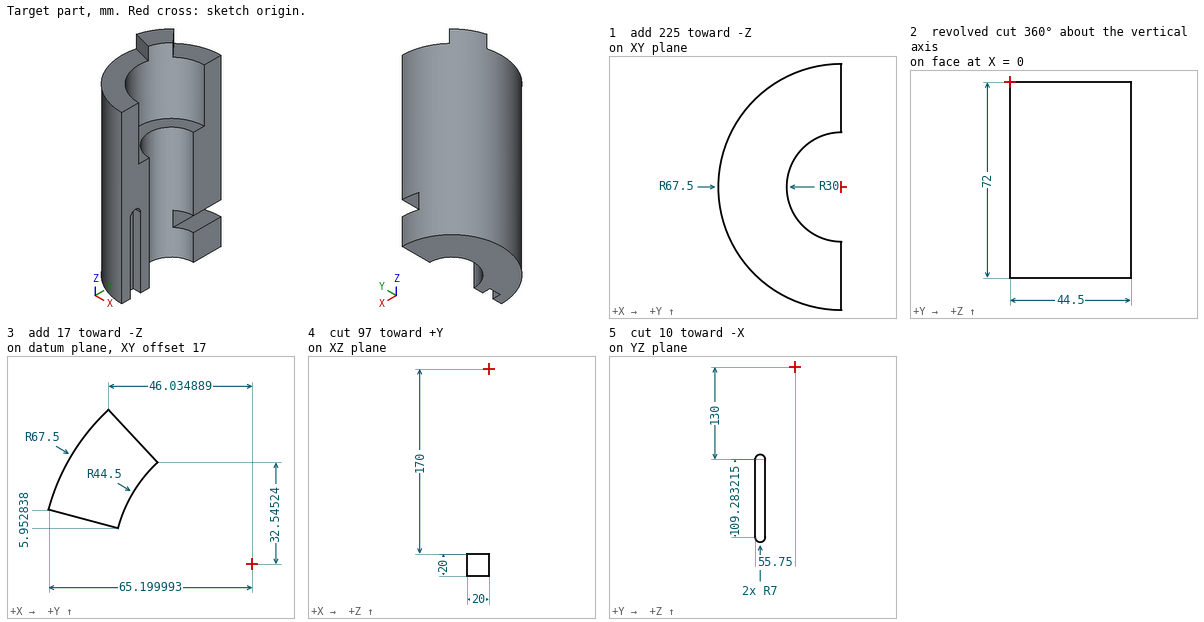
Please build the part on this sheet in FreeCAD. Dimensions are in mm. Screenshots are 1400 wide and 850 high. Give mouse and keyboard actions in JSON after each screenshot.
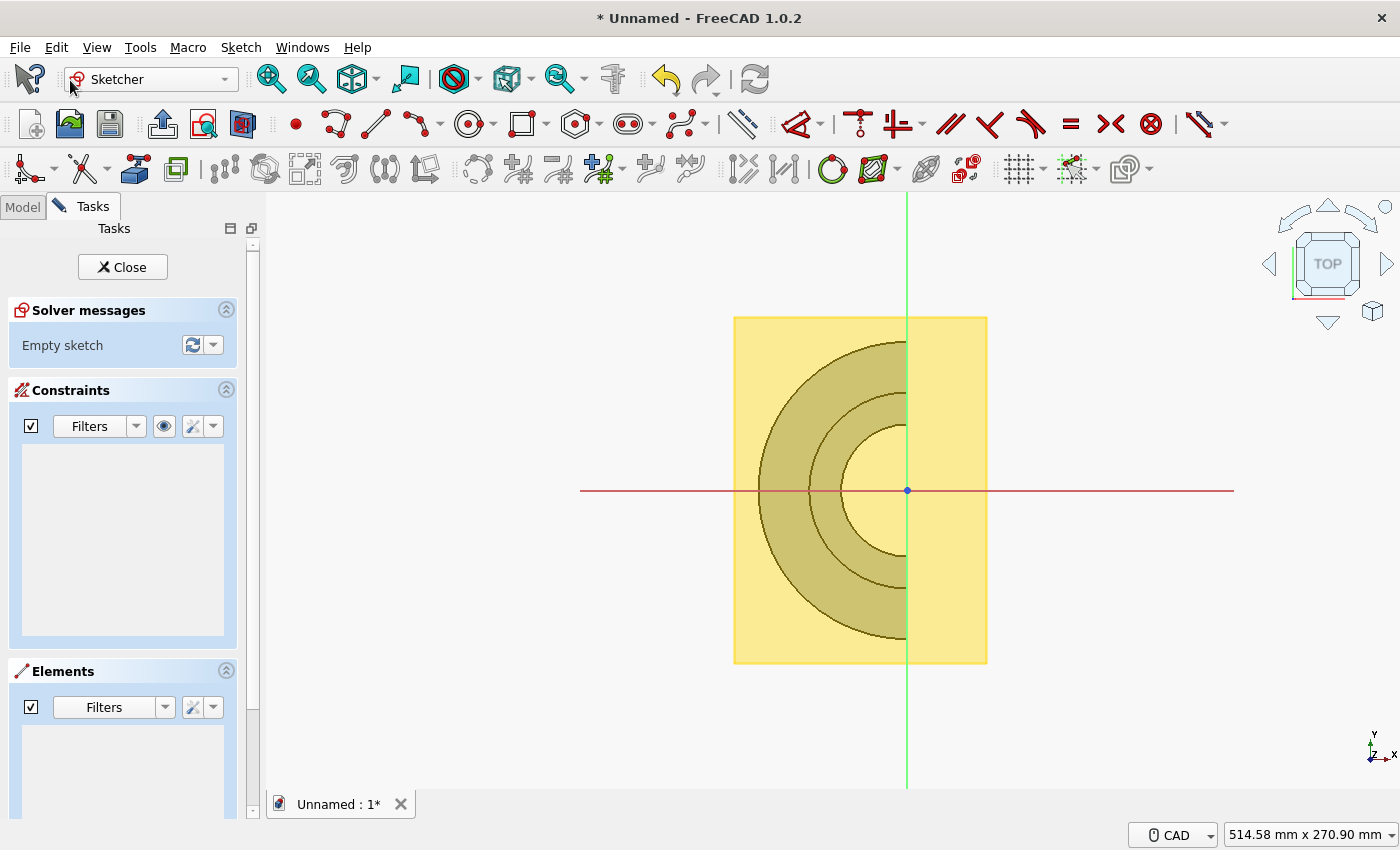
{"action": "scroll", "coordinate": [866, 413], "scroll_direction": "up", "scroll_amount": 6}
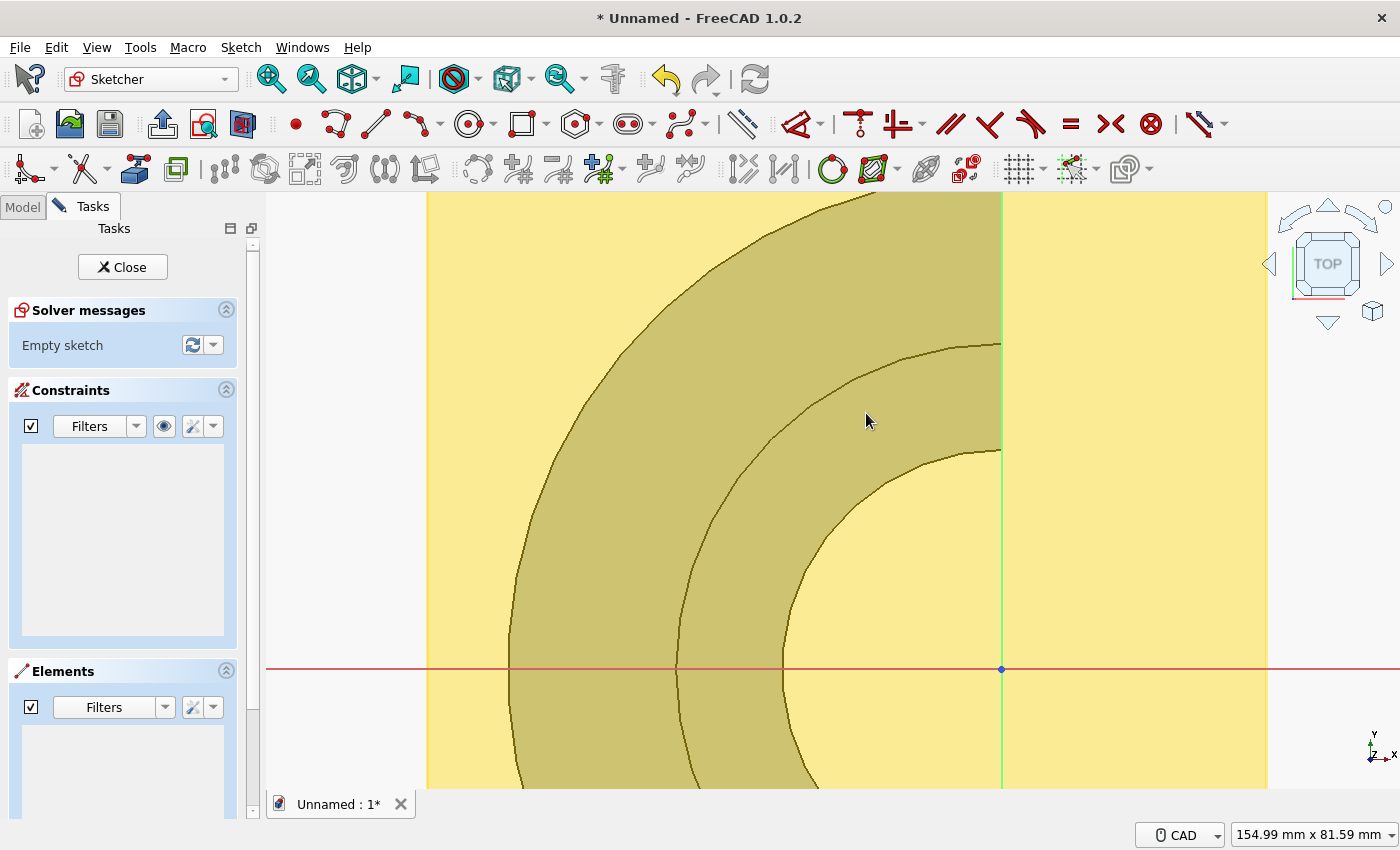
{"action": "key", "text": "g l"}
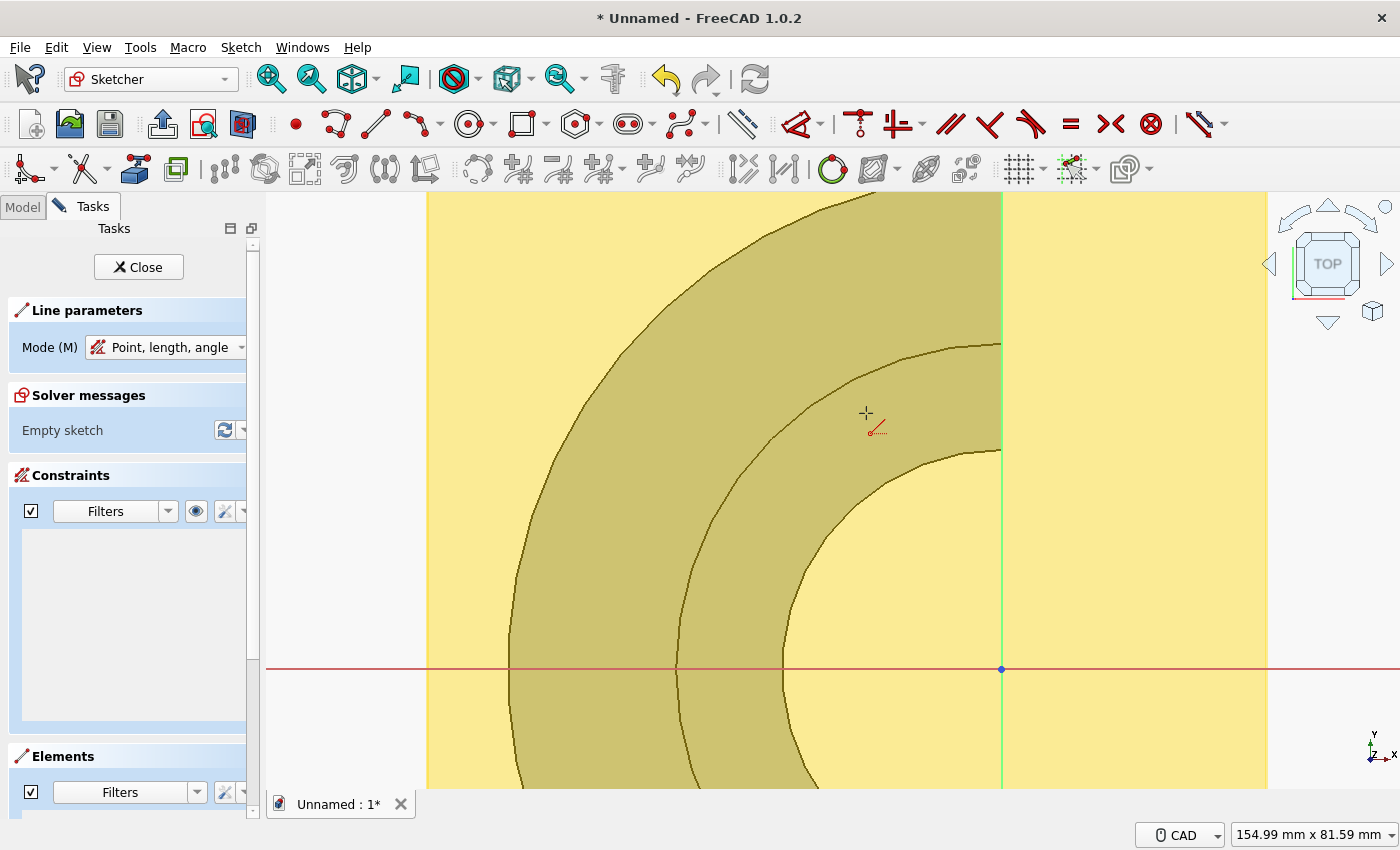
{"action": "left_click", "coordinate": [780, 431]}
{"action": "left_click", "coordinate": [665, 308]}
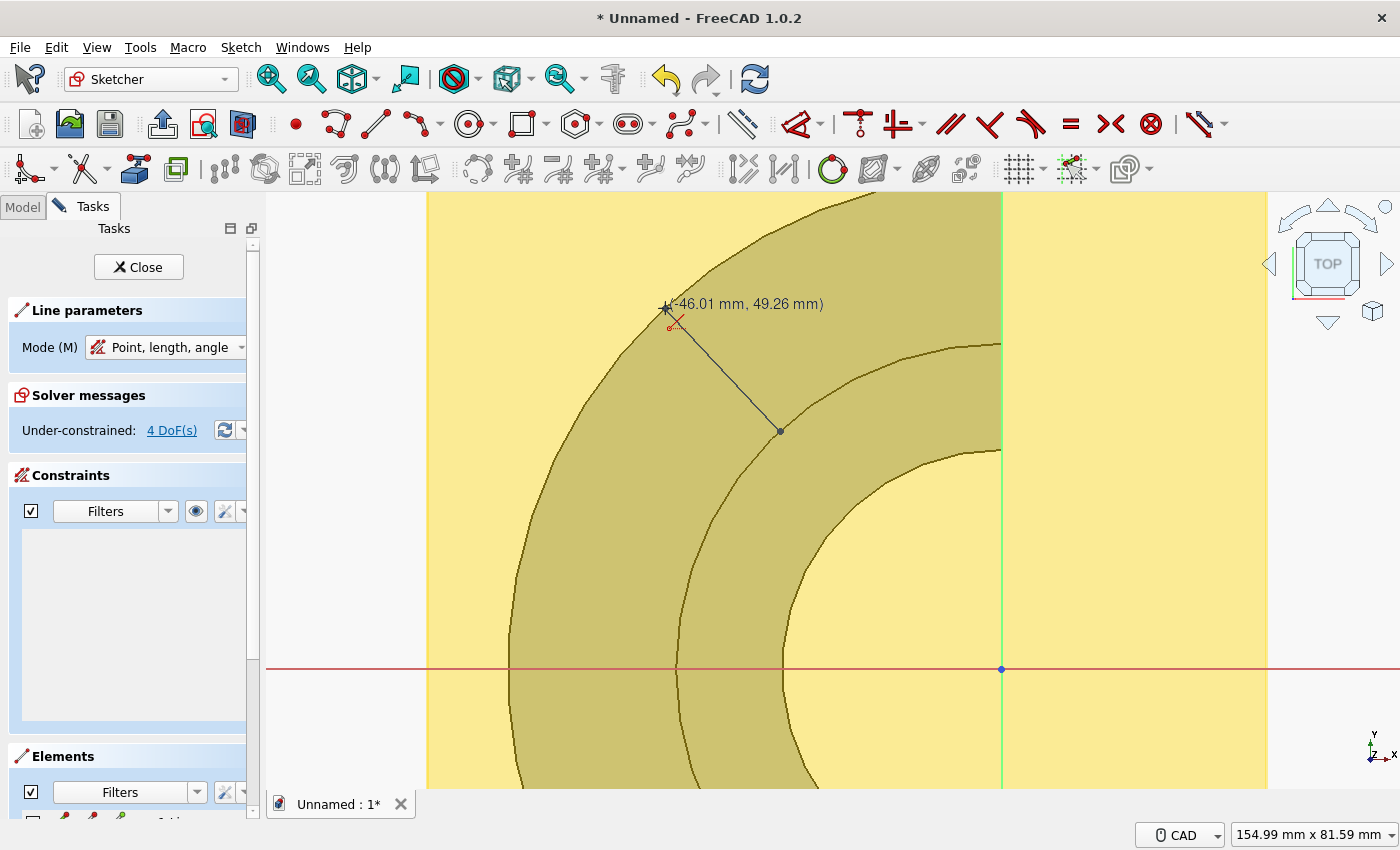
{"action": "left_click", "coordinate": [525, 542]}
{"action": "left_click", "coordinate": [687, 585]}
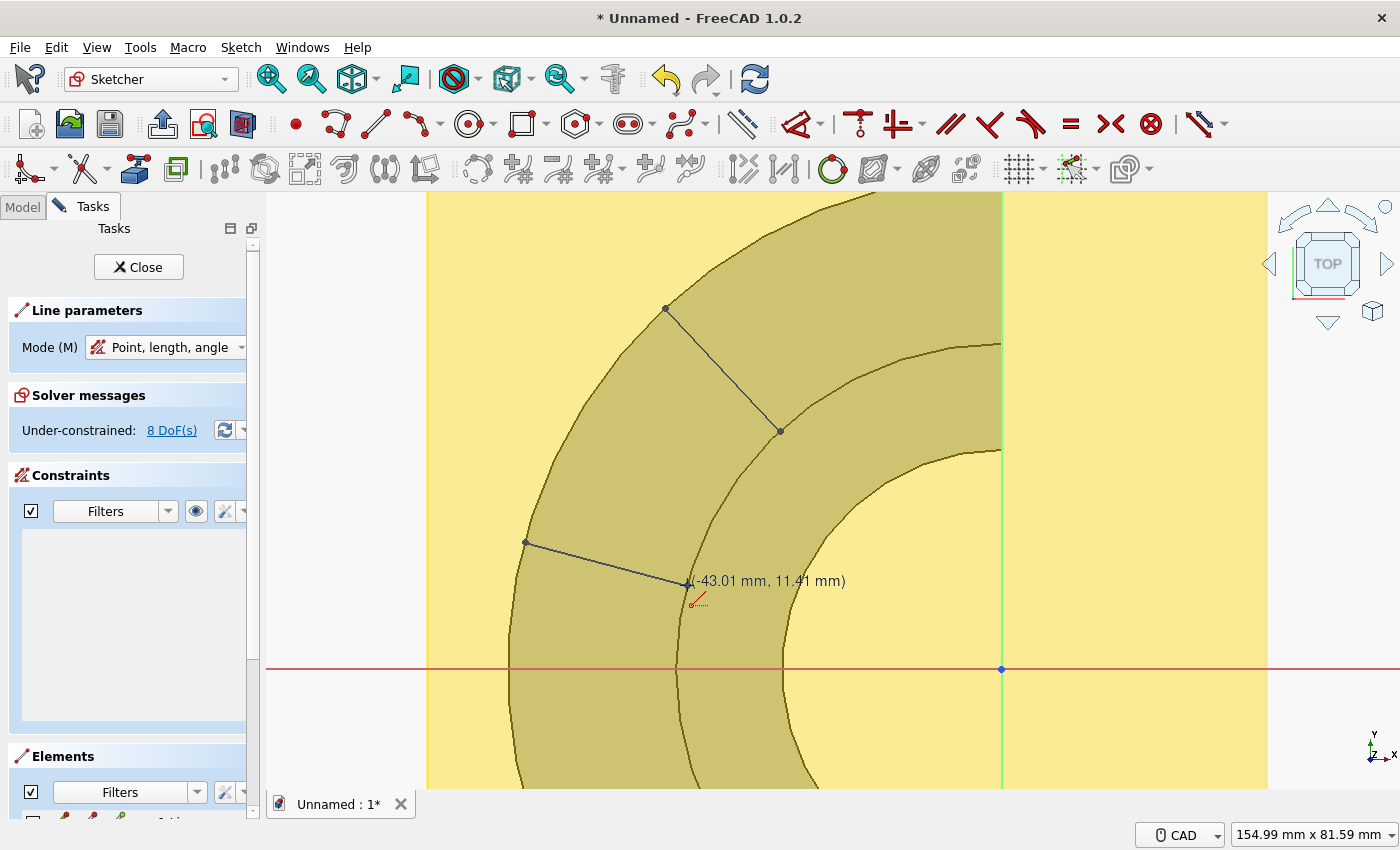
{"action": "key", "text": "g 3 a"}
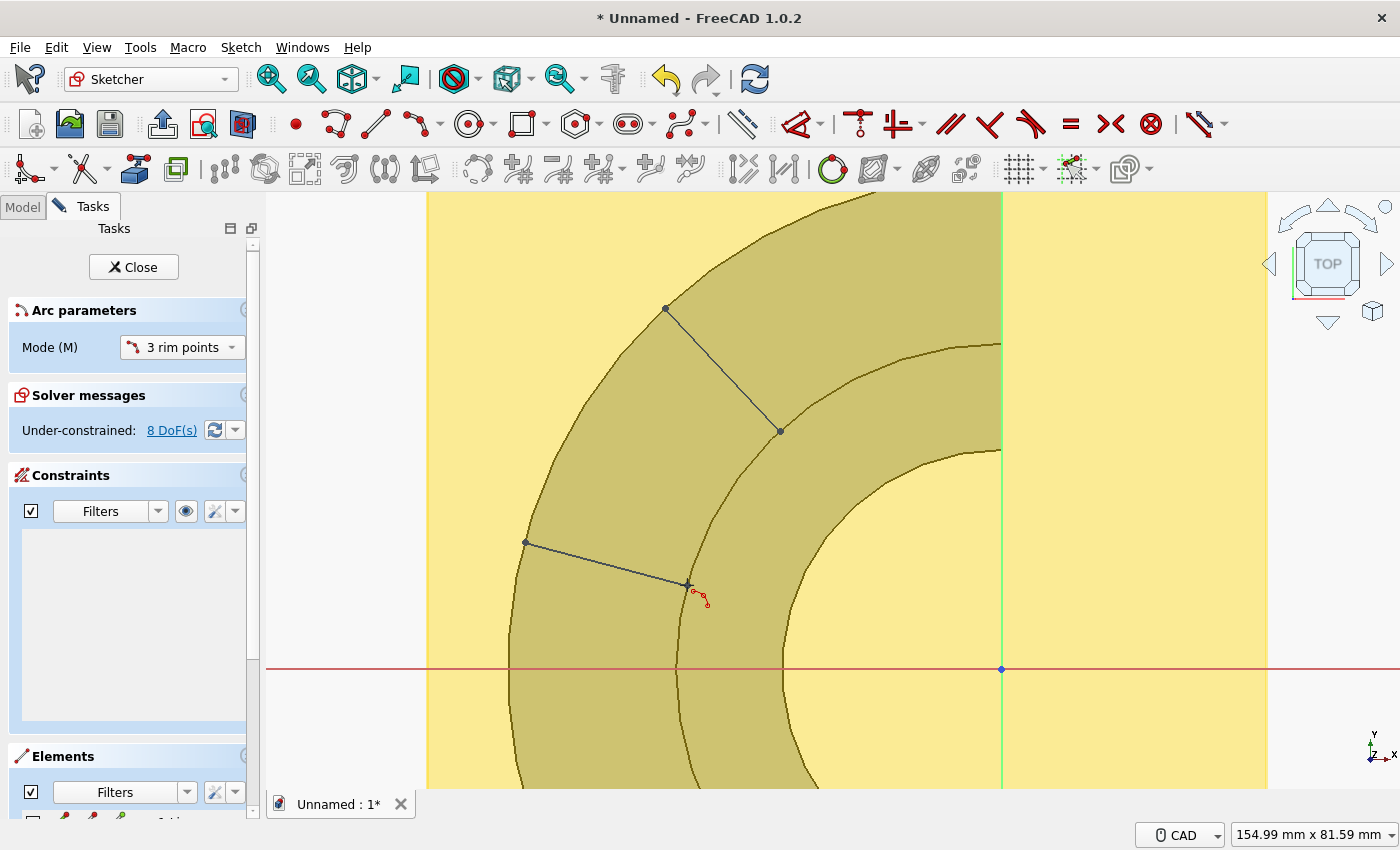
{"action": "left_click", "coordinate": [665, 309]}
{"action": "left_click", "coordinate": [525, 543]}
{"action": "left_click", "coordinate": [578, 415]}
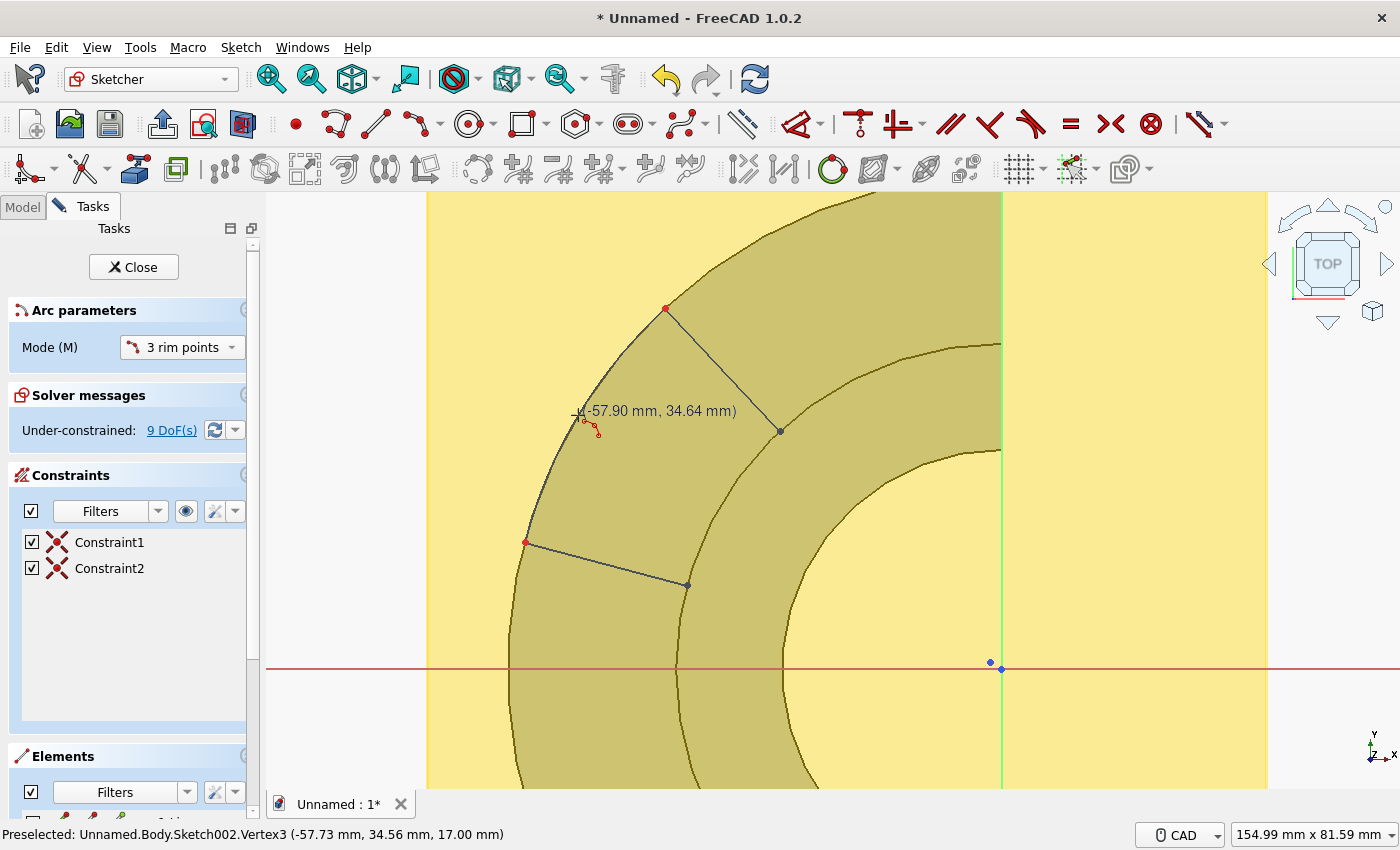
{"action": "left_click", "coordinate": [687, 586]}
{"action": "left_click", "coordinate": [780, 432]}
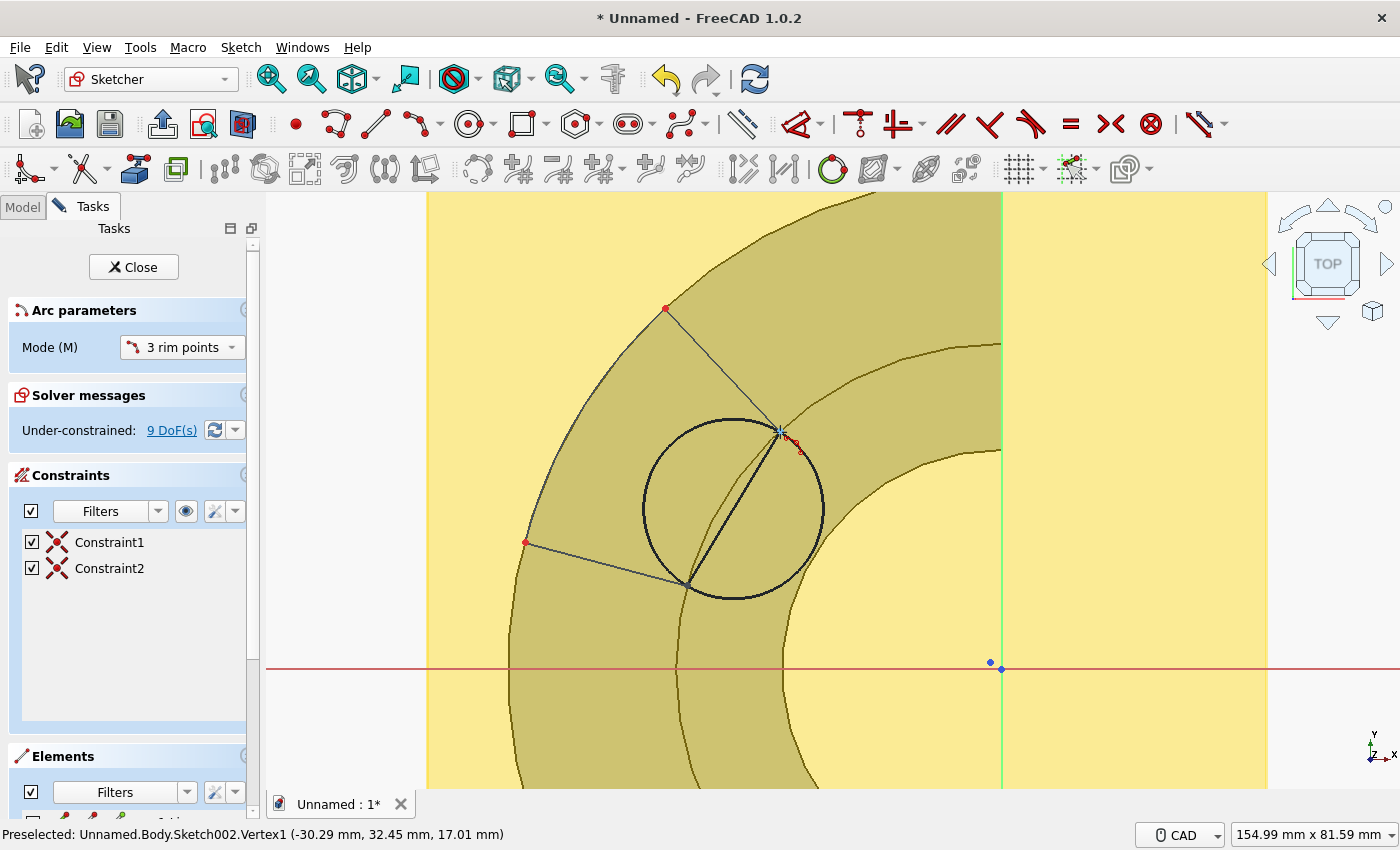
{"action": "scroll", "coordinate": [723, 502], "scroll_direction": "up", "scroll_amount": 2}